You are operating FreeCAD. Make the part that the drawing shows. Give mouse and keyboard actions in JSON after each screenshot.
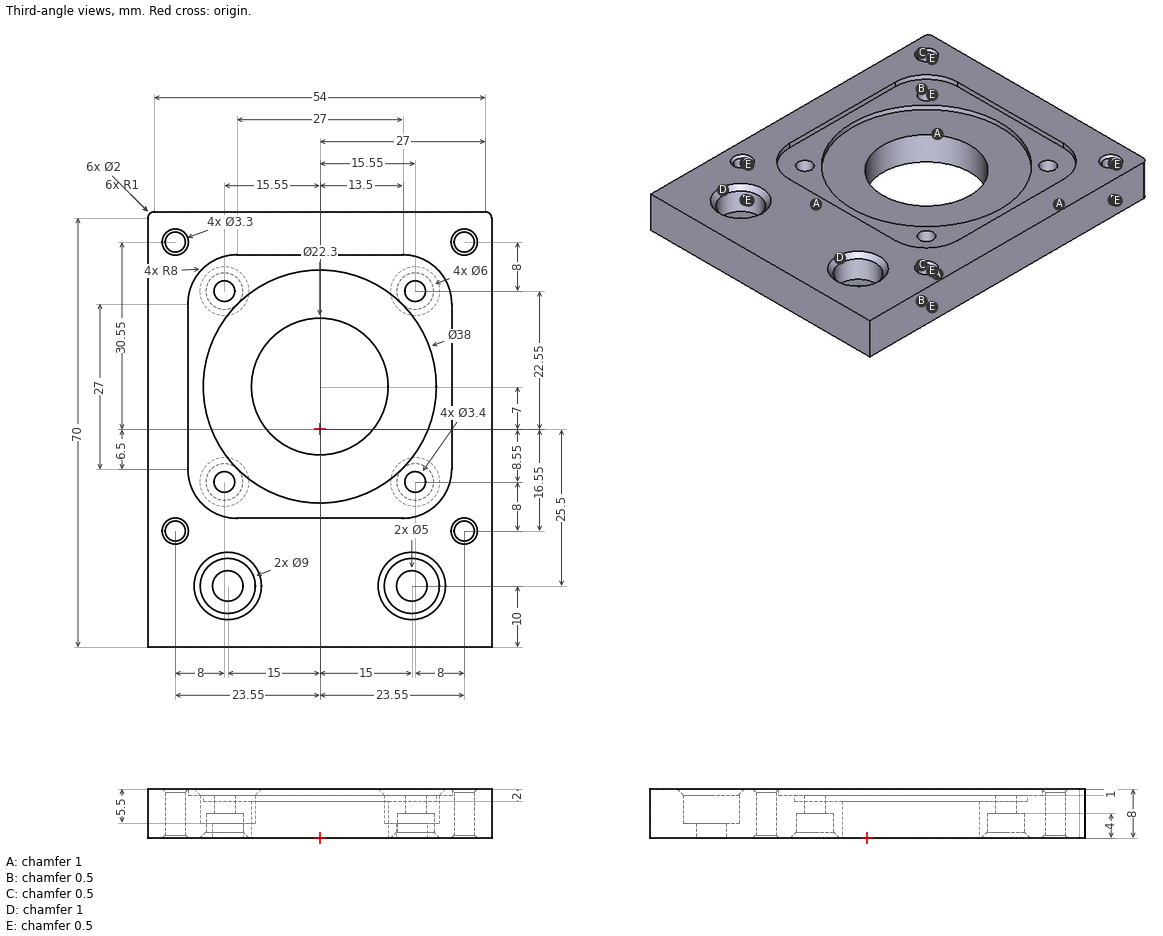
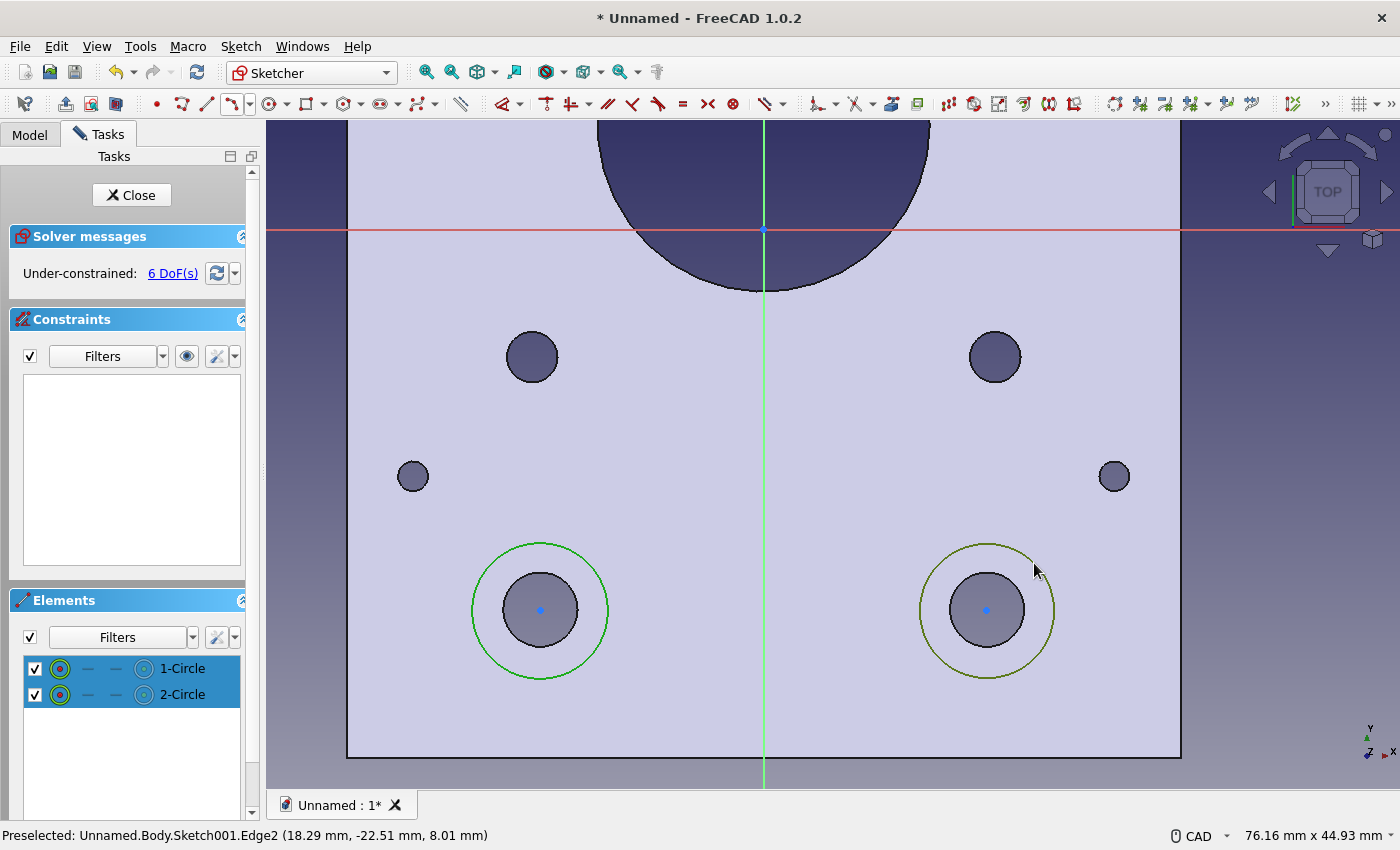
{"action": "key", "text": "e"}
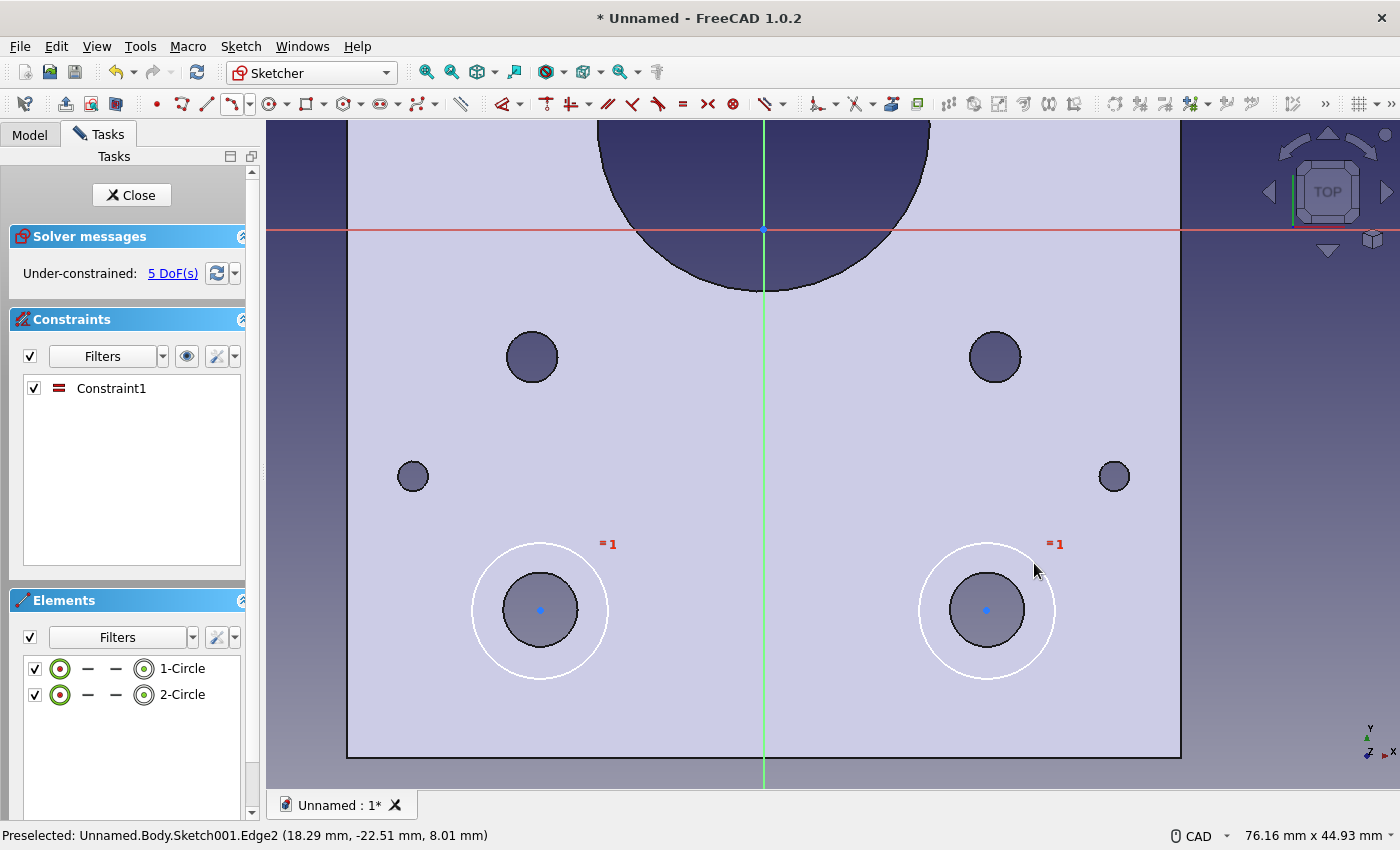
{"action": "left_click", "coordinate": [502, 104]}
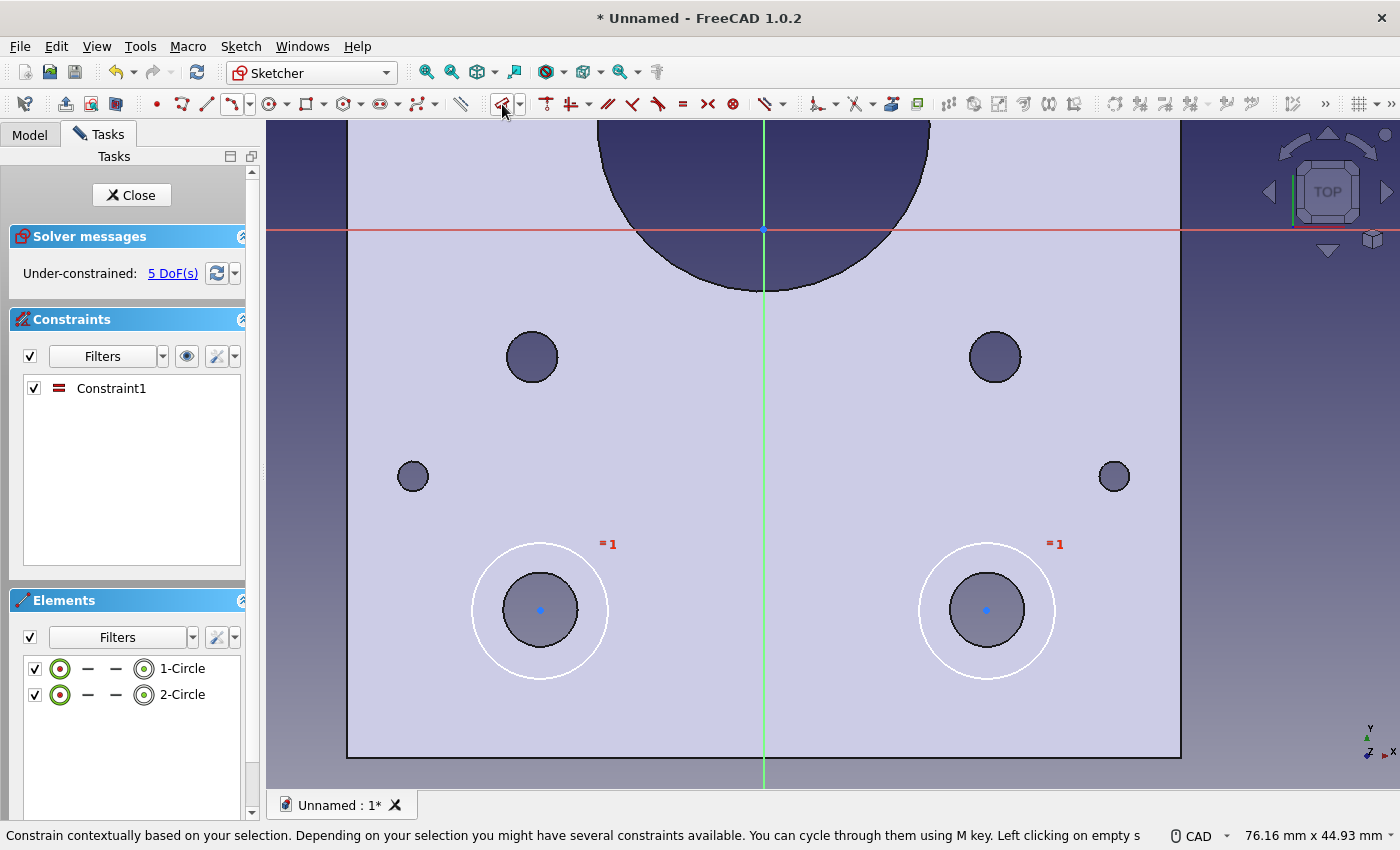
{"action": "left_click", "coordinate": [588, 563]}
{"action": "left_click", "coordinate": [611, 540]}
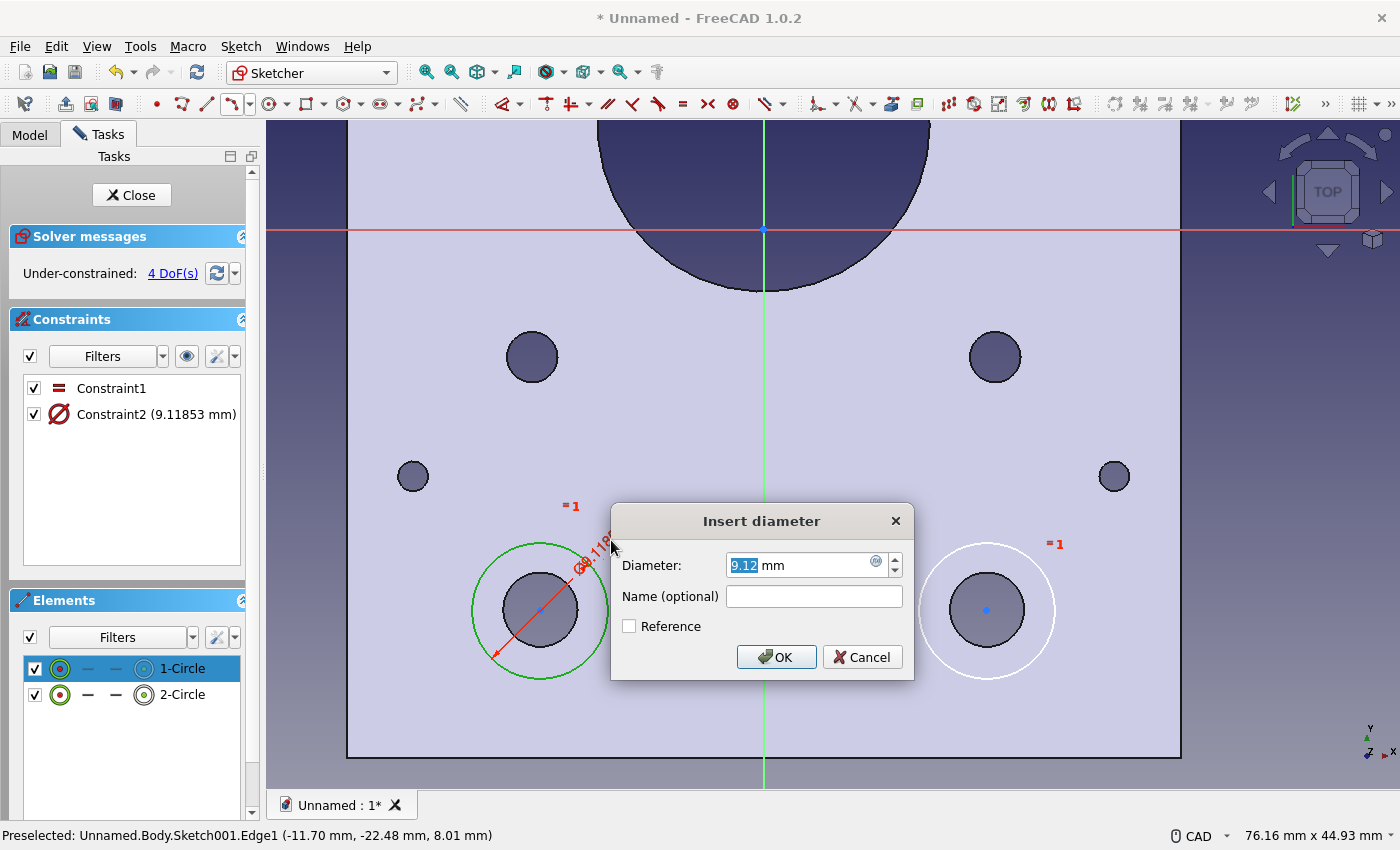
{"action": "type", "text": "9"}
{"action": "key", "text": "Return"}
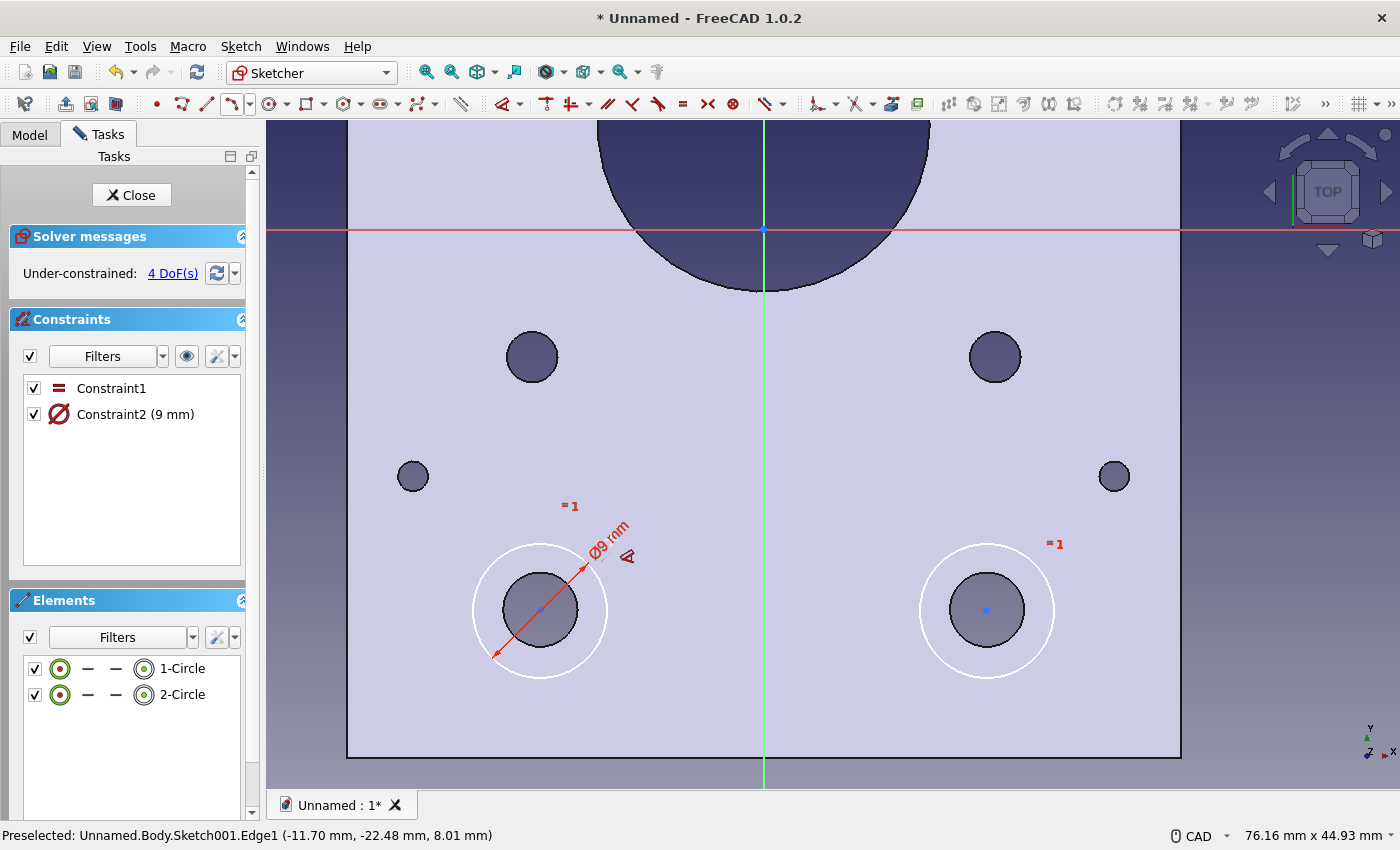
{"action": "left_click", "coordinate": [540, 611]}
{"action": "left_click", "coordinate": [652, 196]}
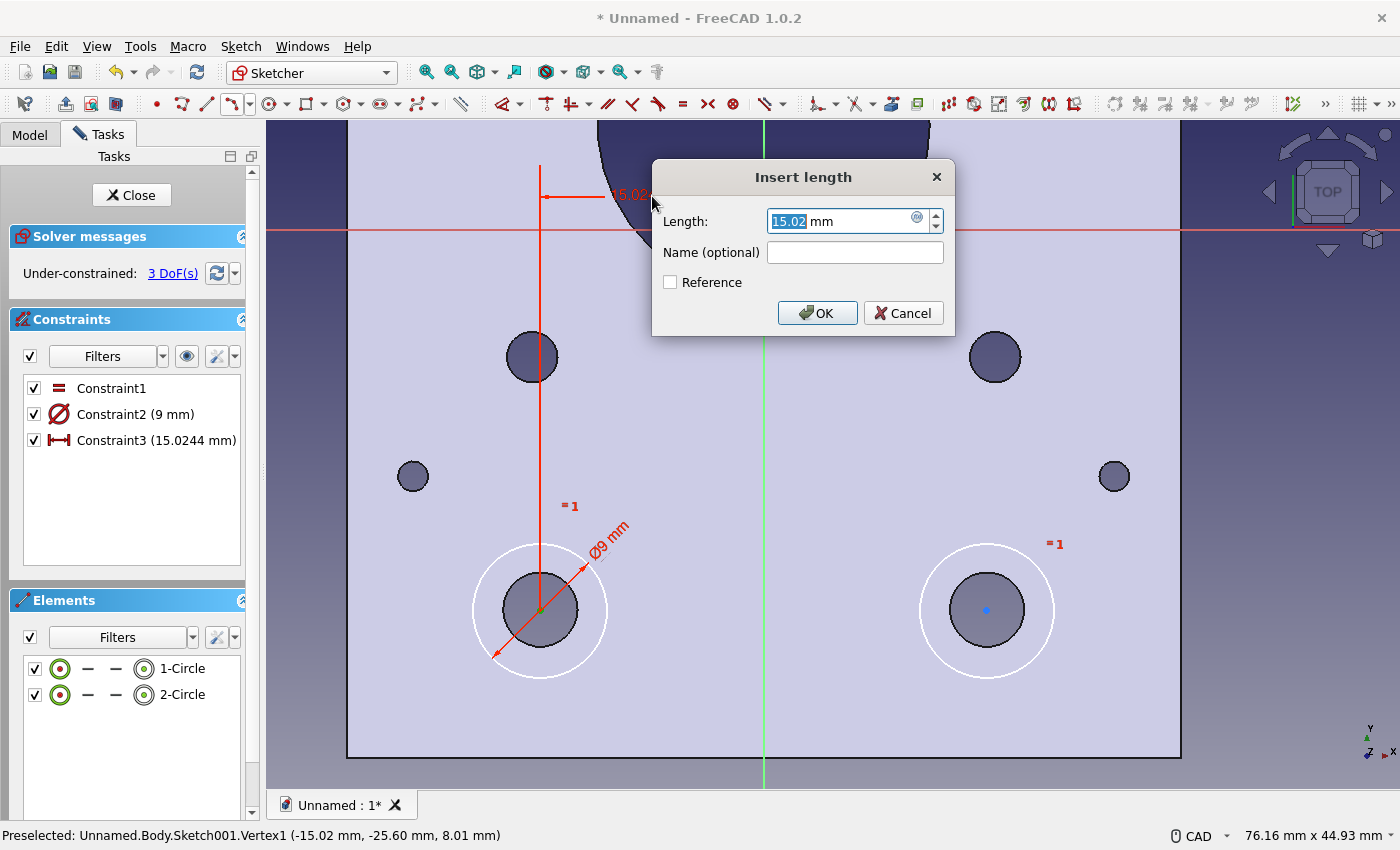
{"action": "type", "text": "15"}
{"action": "key", "text": "Return"}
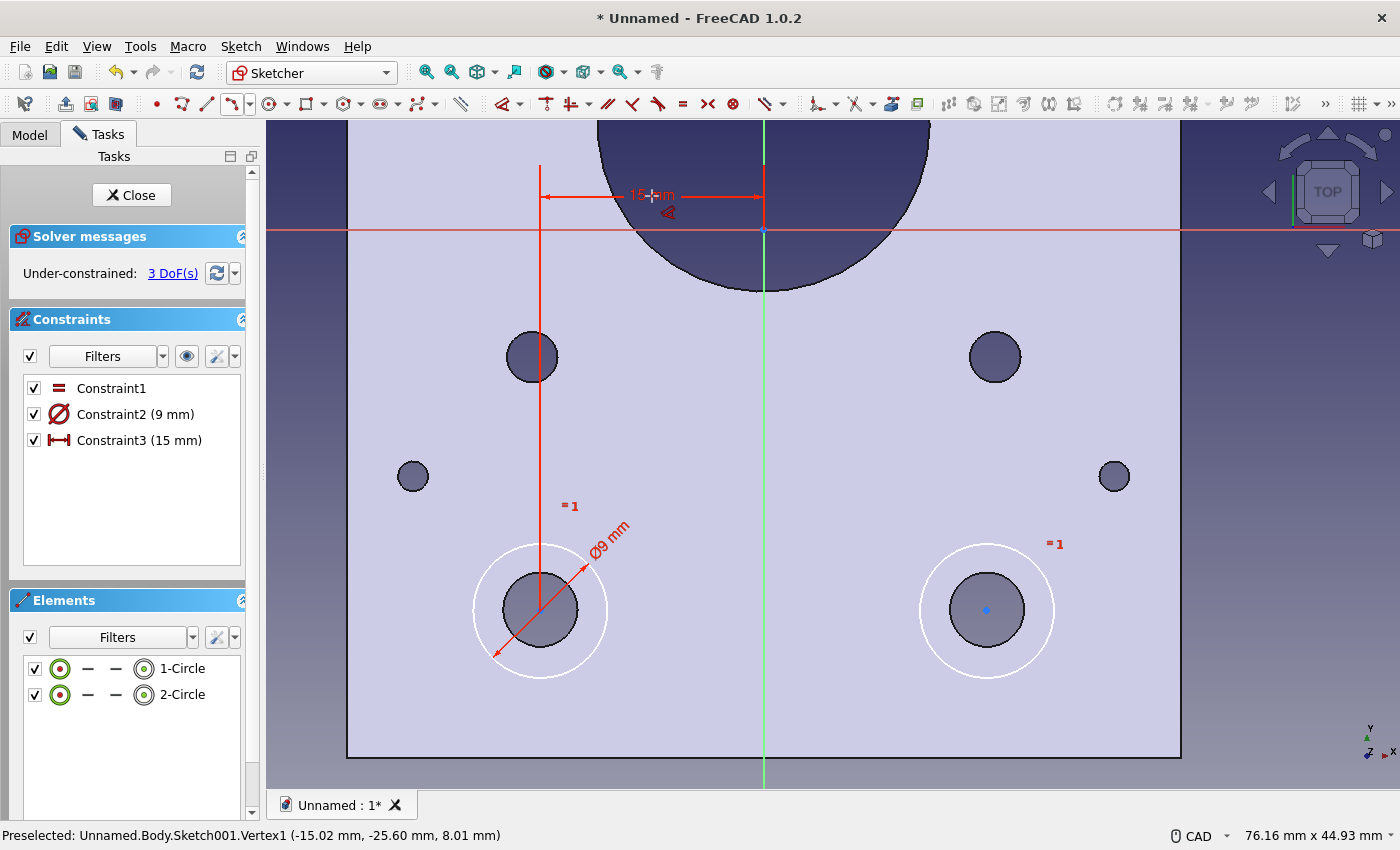
{"action": "left_click", "coordinate": [987, 611]}
{"action": "left_click", "coordinate": [875, 196]}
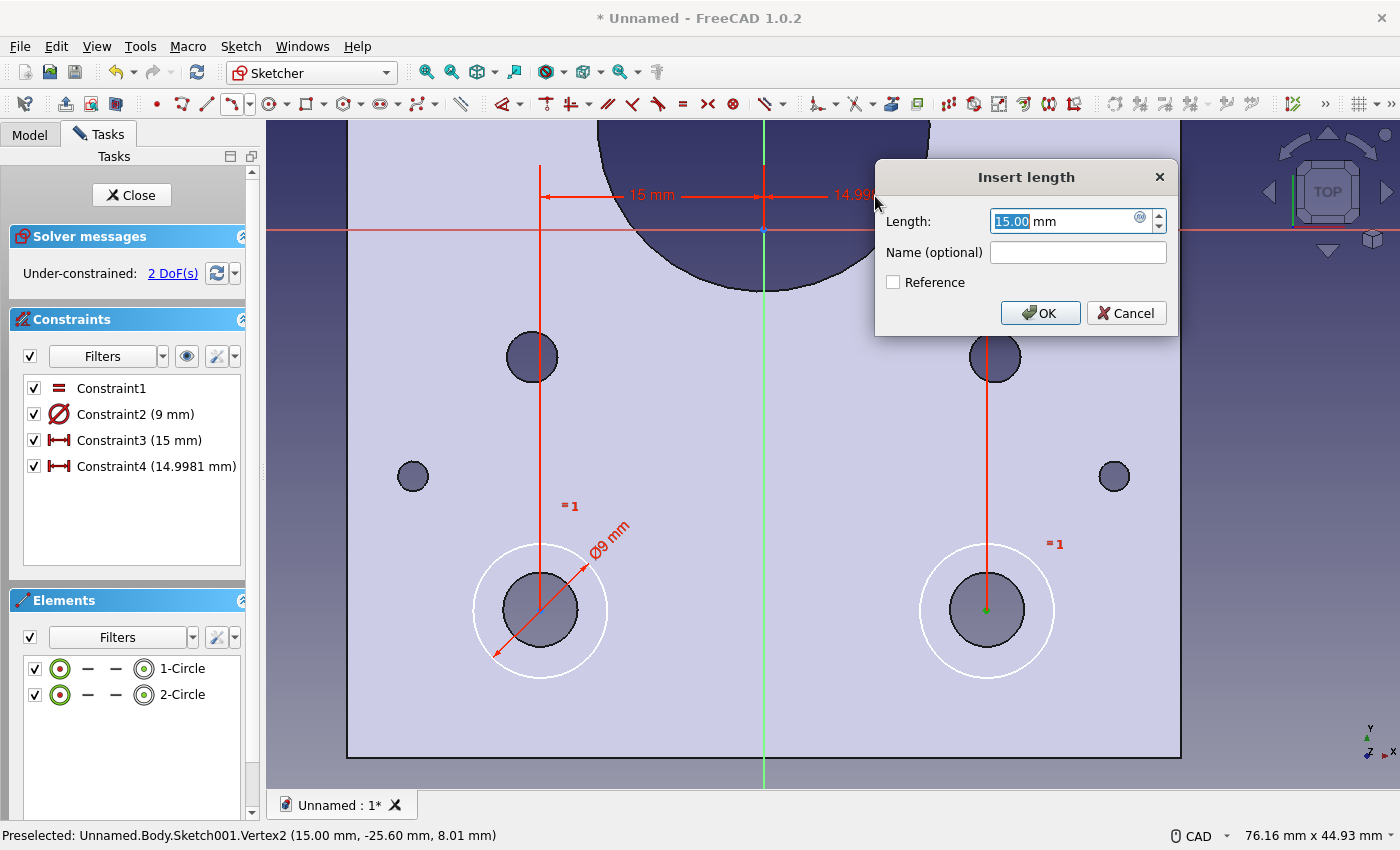
{"action": "type", "text": "15"}
{"action": "key", "text": "Return"}